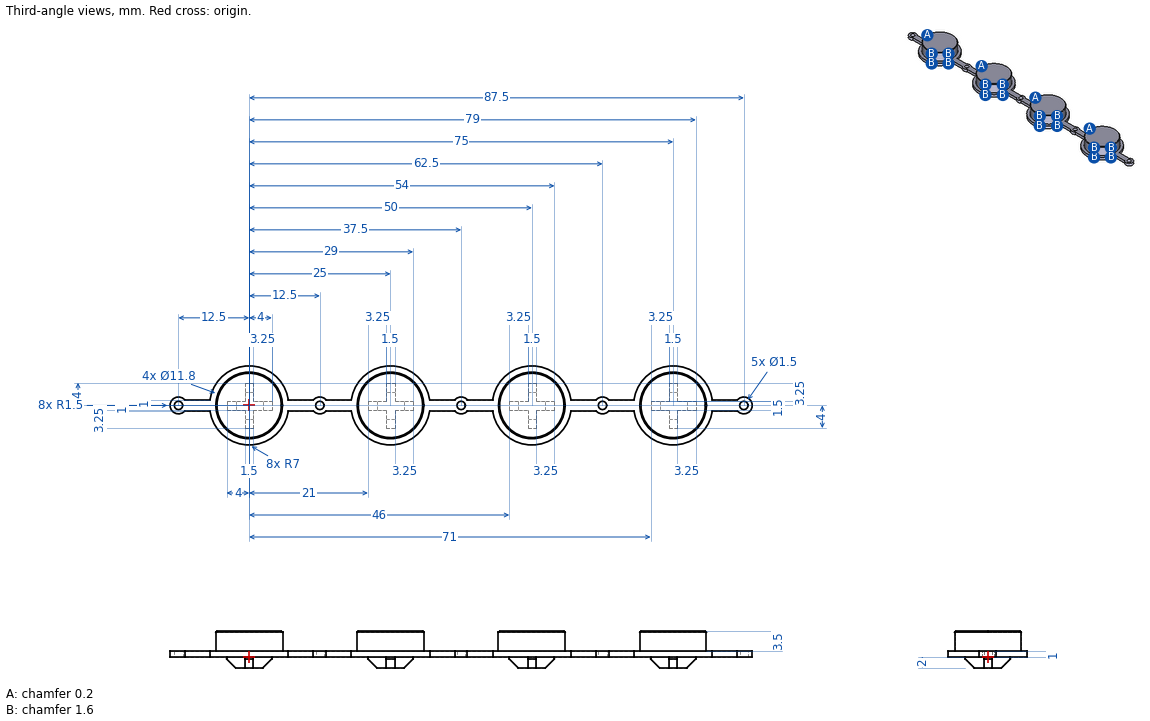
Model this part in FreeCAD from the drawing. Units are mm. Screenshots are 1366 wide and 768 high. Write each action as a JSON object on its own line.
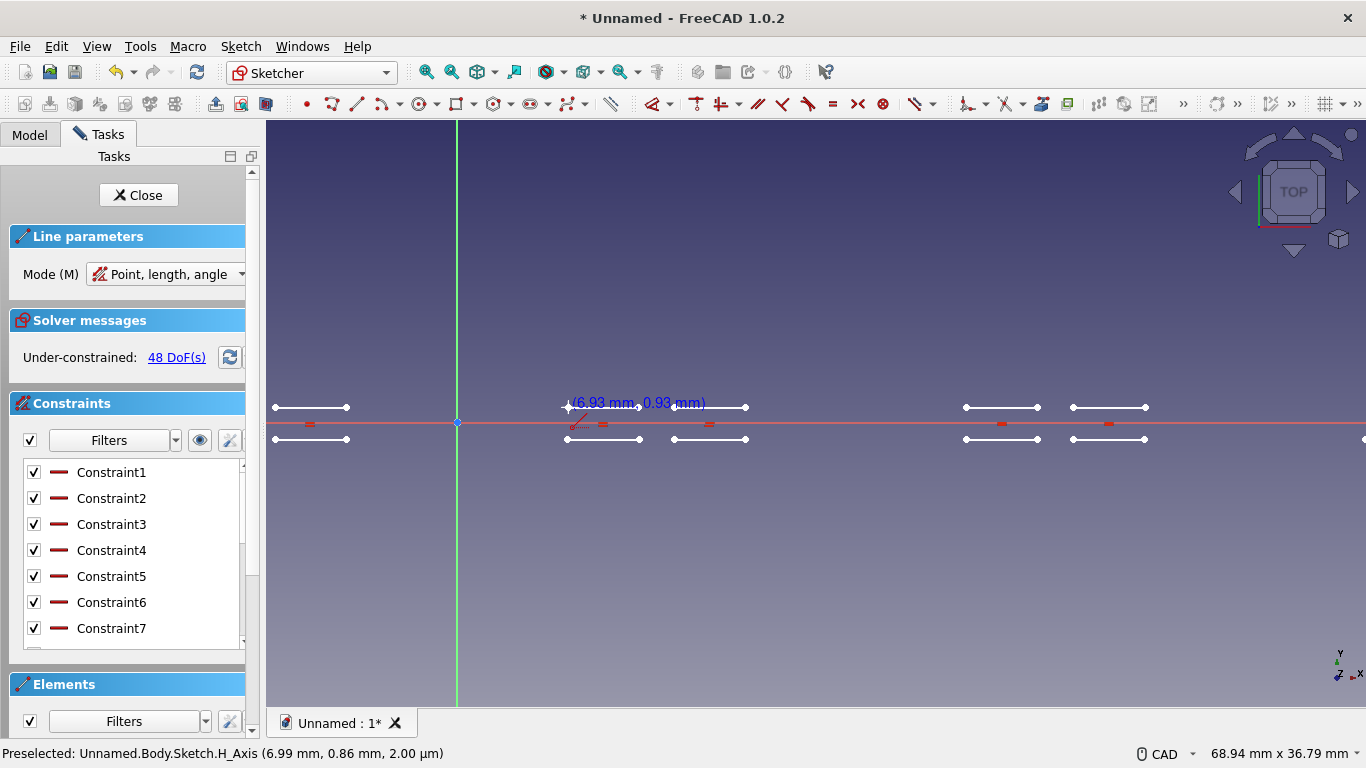
{"action": "key", "text": "g 3 a"}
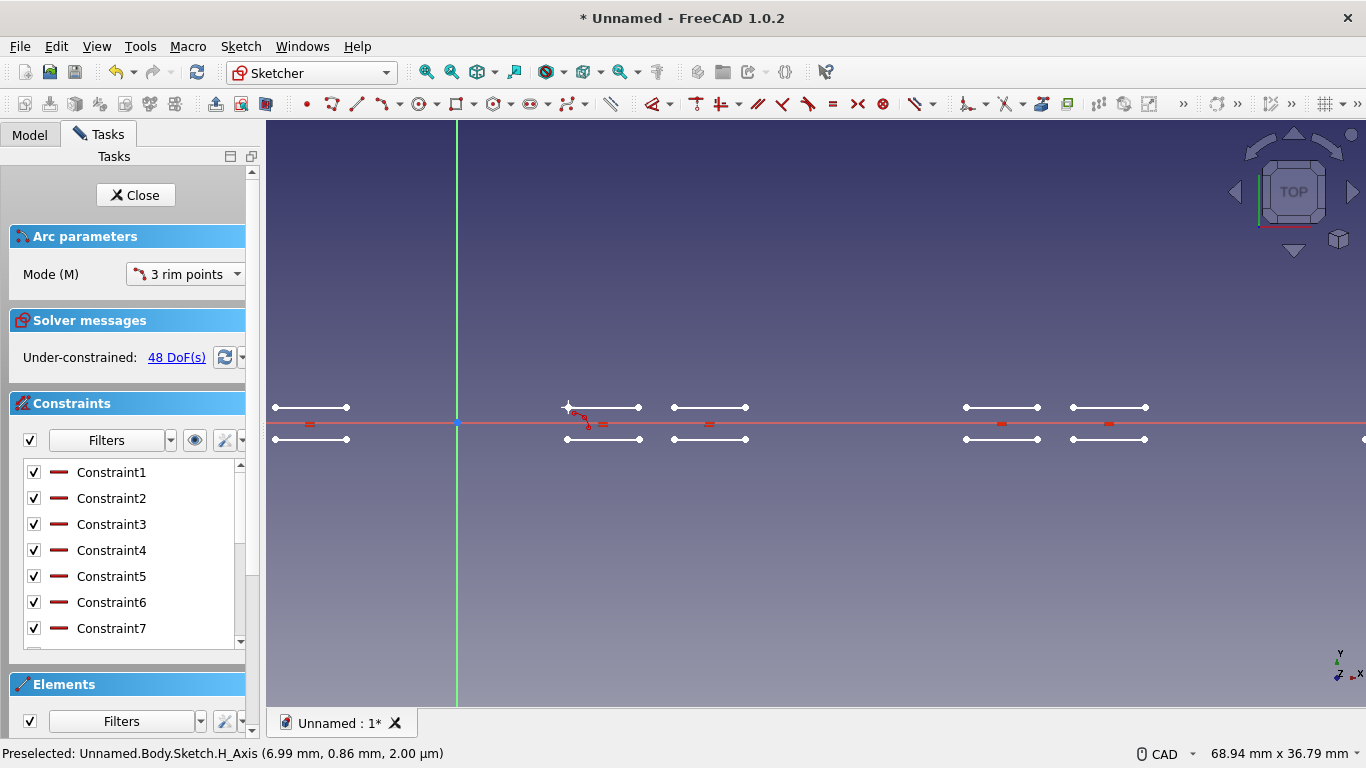
{"action": "scroll", "coordinate": [568, 408], "scroll_direction": "down", "scroll_amount": 5}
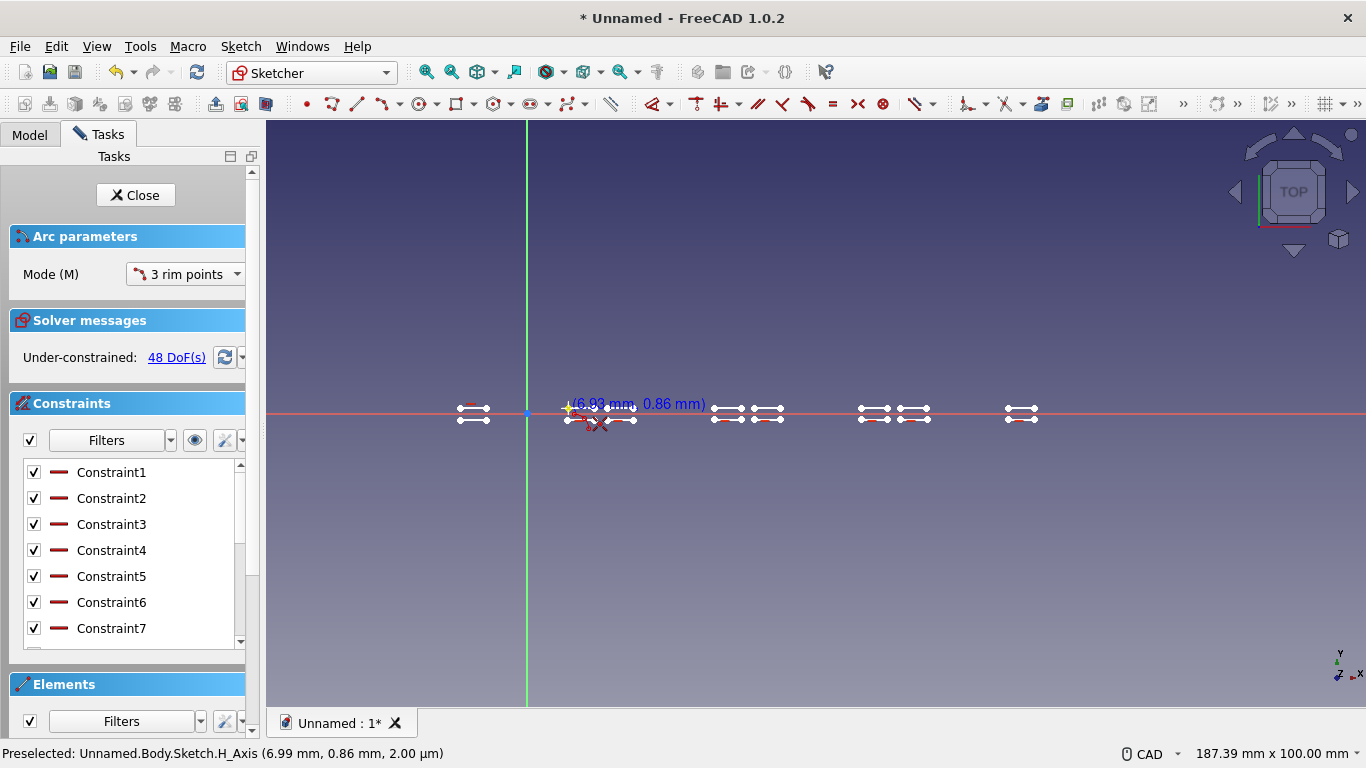
{"action": "scroll", "coordinate": [461, 408], "scroll_direction": "up", "scroll_amount": 5}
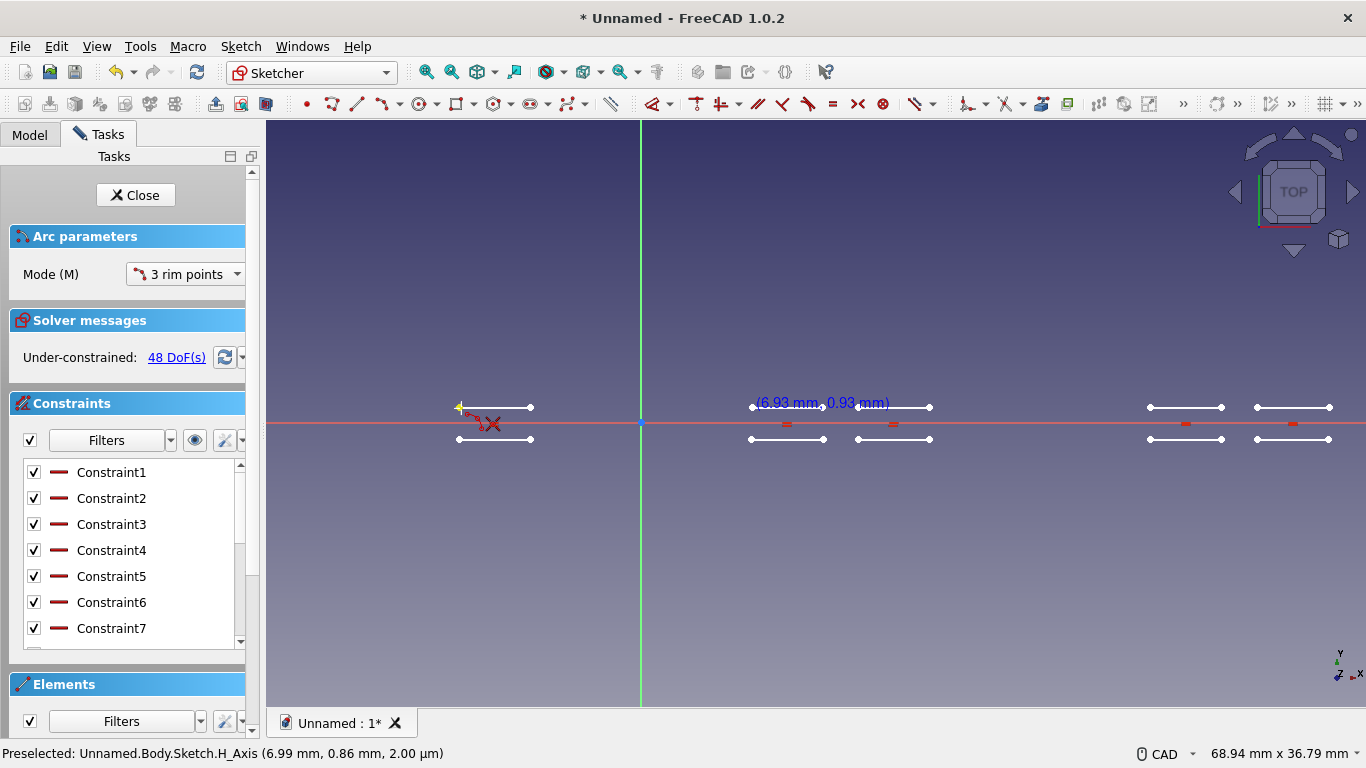
{"action": "left_click", "coordinate": [459, 408]}
{"action": "left_click", "coordinate": [459, 440]}
{"action": "left_click", "coordinate": [428, 403]}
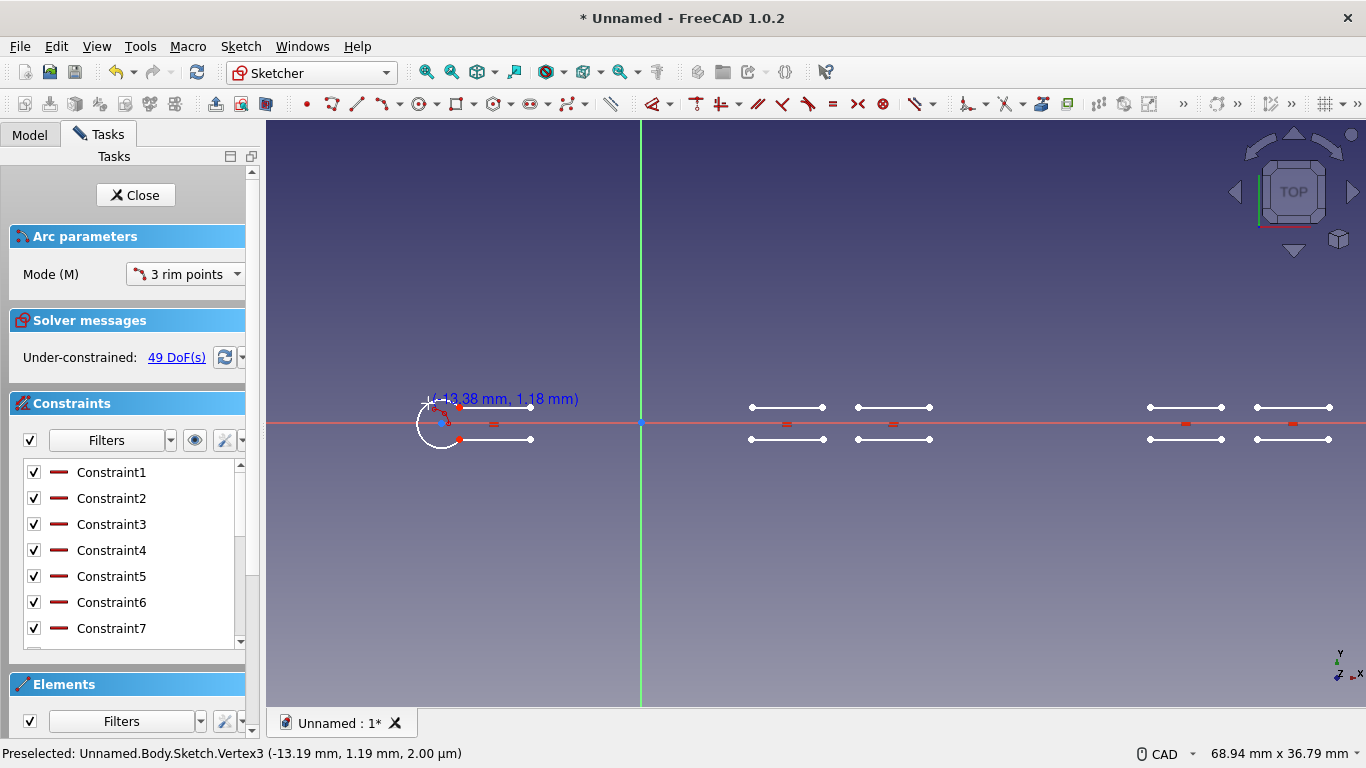
{"action": "left_click", "coordinate": [530, 440]}
{"action": "left_click", "coordinate": [751, 440]}
{"action": "left_click", "coordinate": [581, 517]}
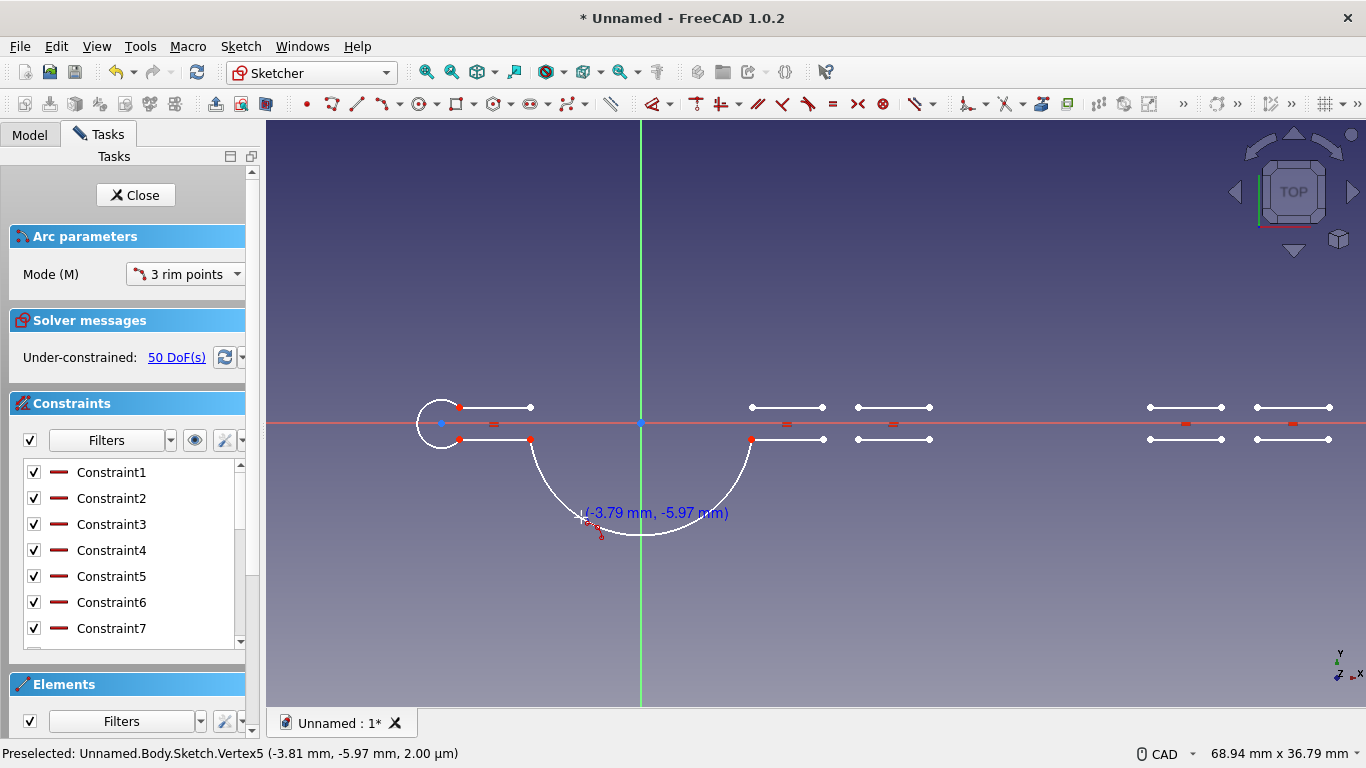
{"action": "left_click", "coordinate": [823, 440]}
{"action": "left_click", "coordinate": [858, 440]}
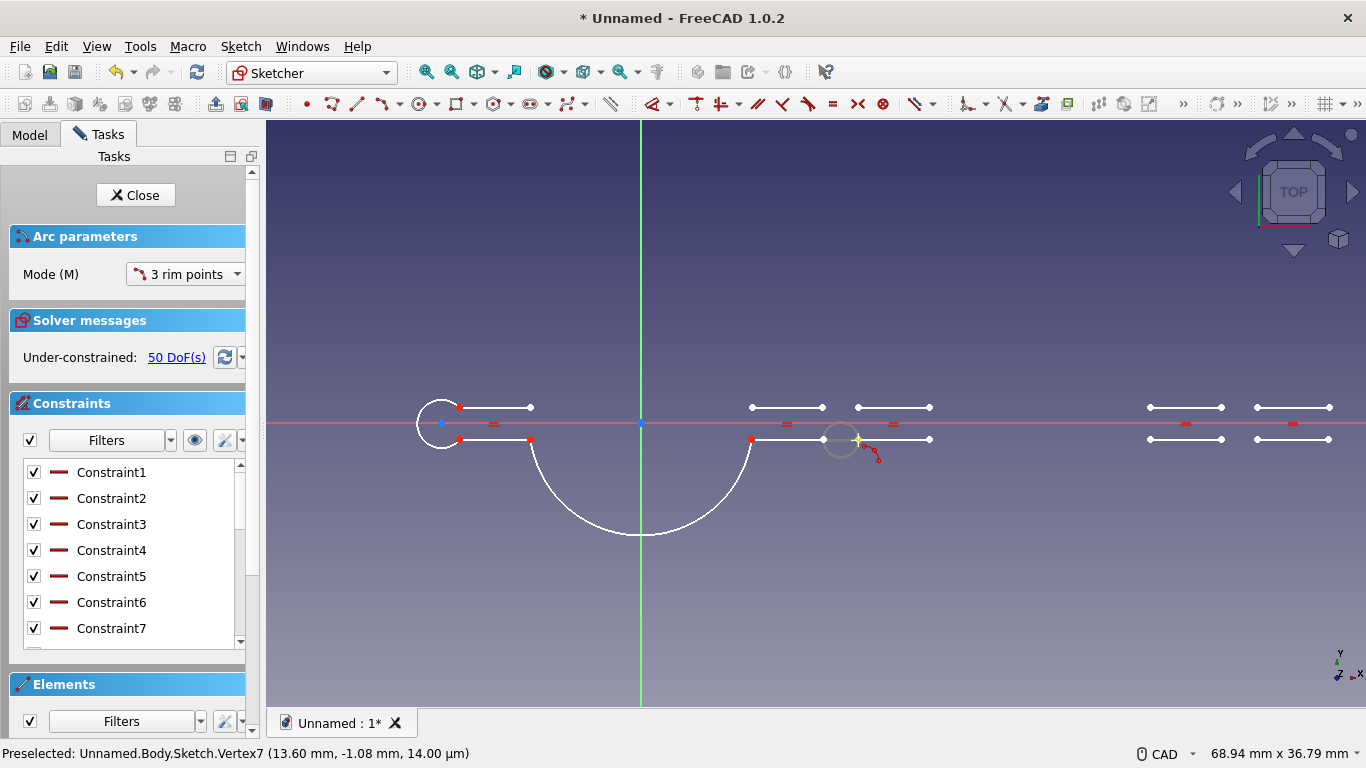
{"action": "scroll", "coordinate": [841, 447], "scroll_direction": "up", "scroll_amount": 4}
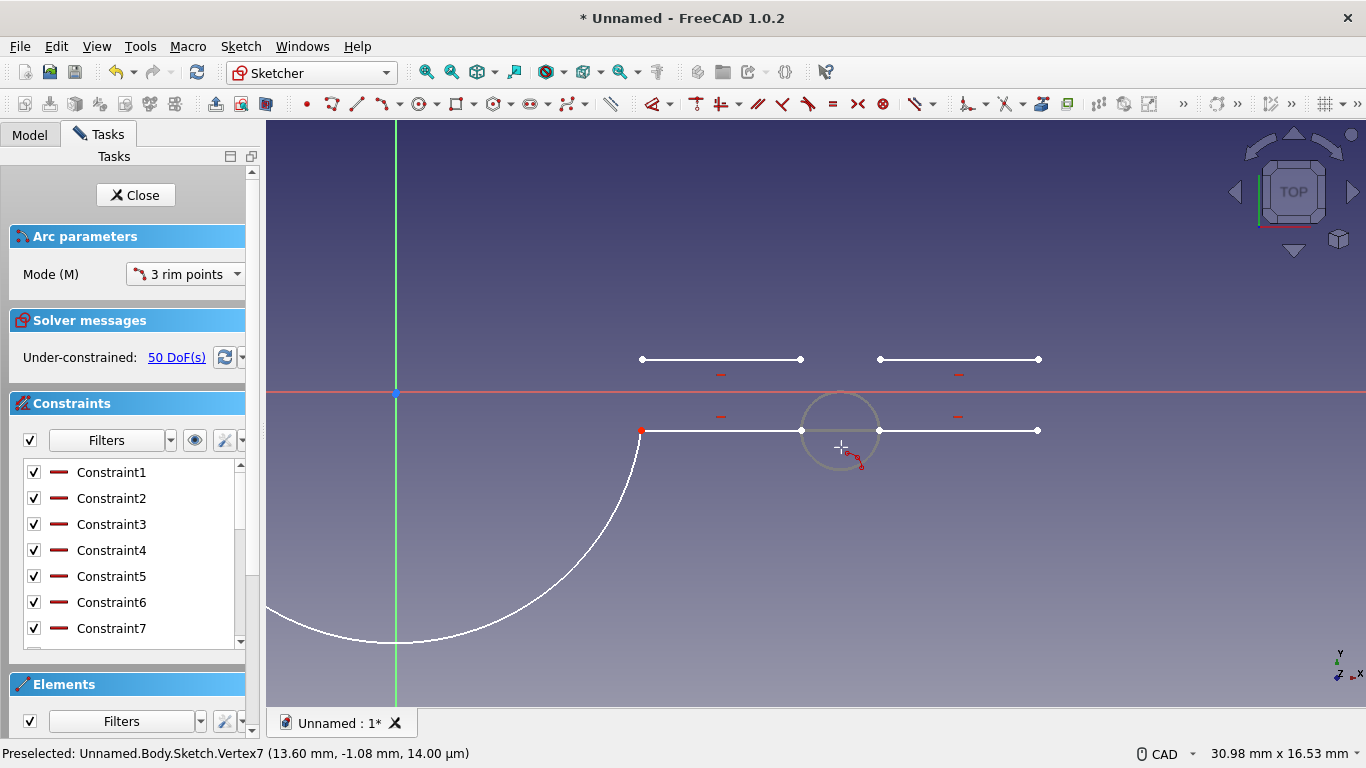
{"action": "left_click", "coordinate": [840, 446]}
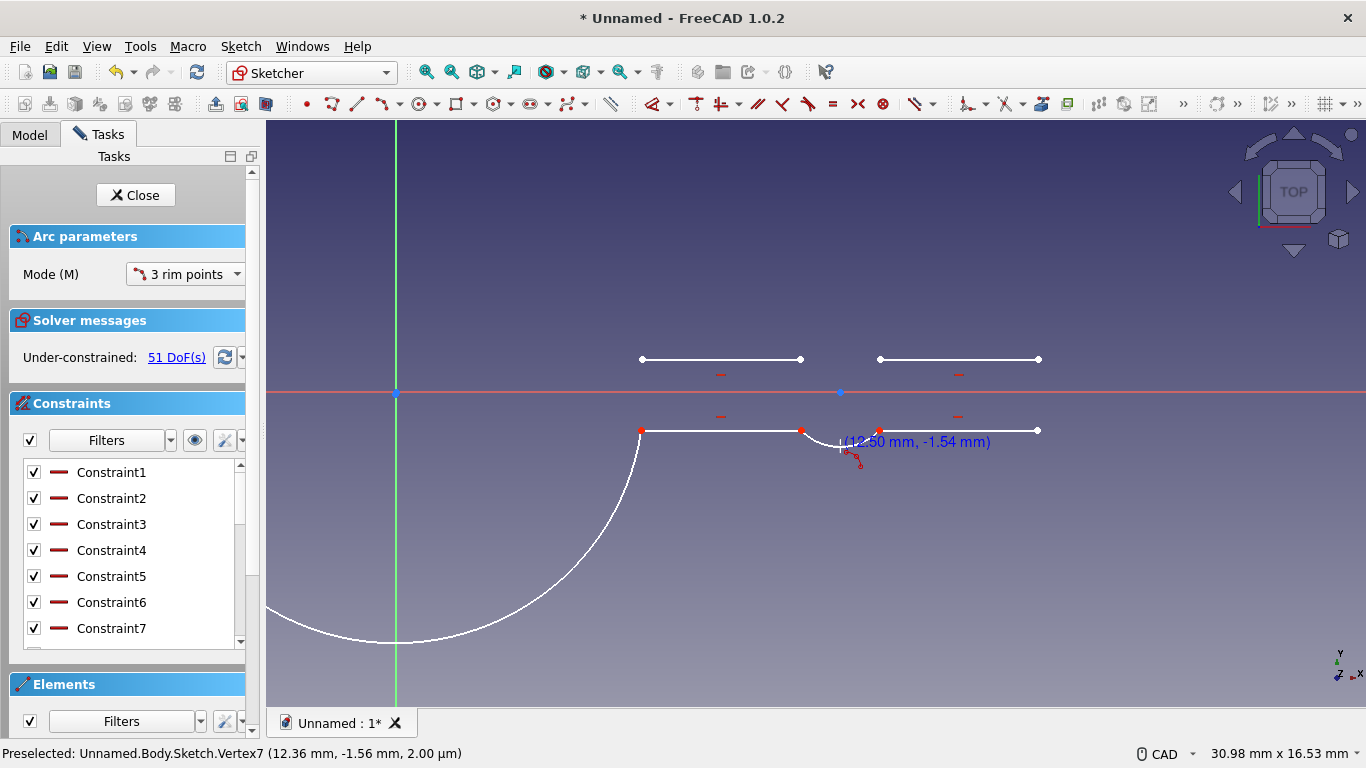
{"action": "left_click", "coordinate": [1037, 431]}